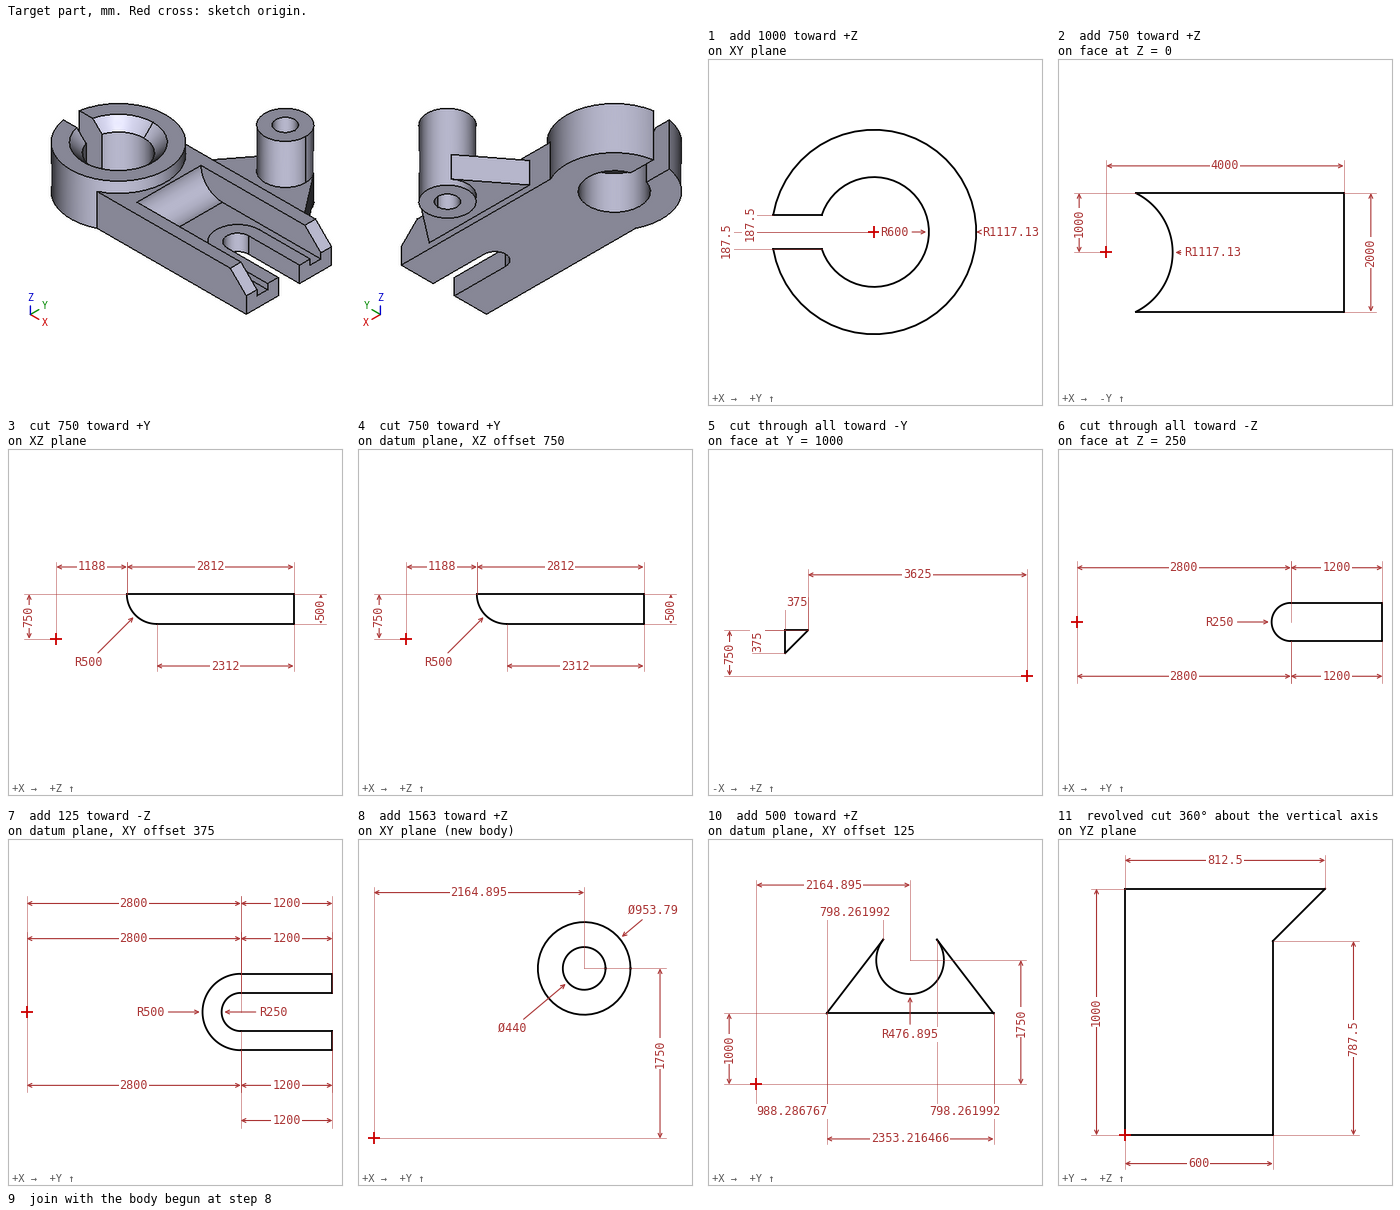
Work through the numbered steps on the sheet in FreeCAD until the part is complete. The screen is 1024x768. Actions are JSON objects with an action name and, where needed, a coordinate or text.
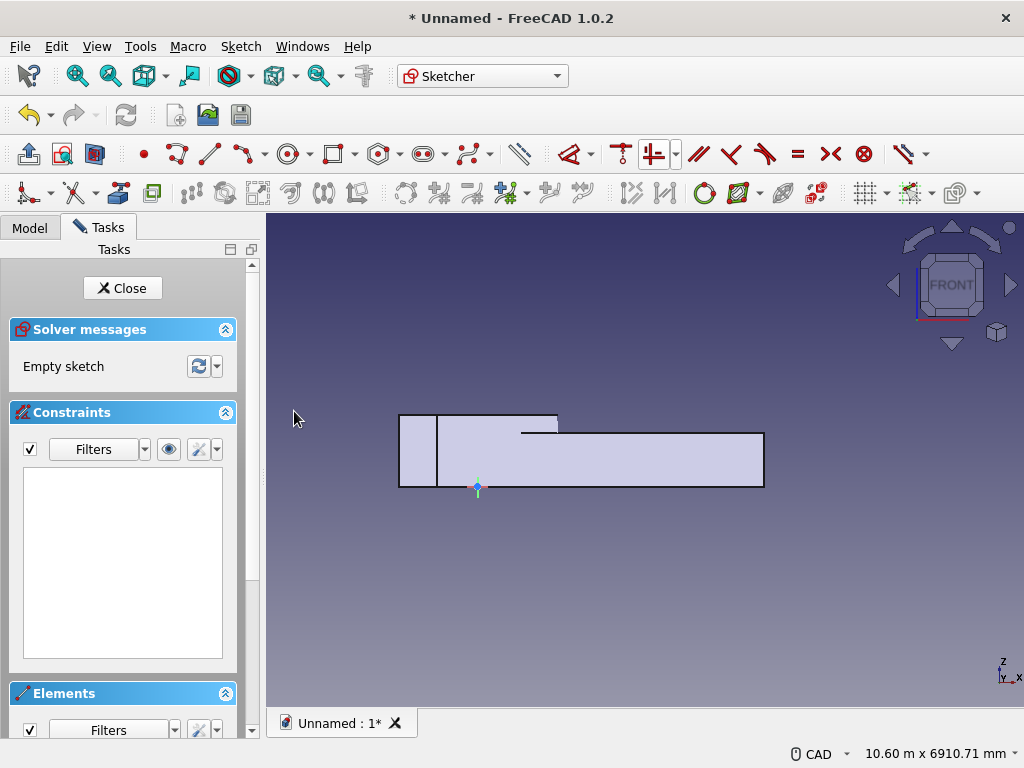
{"action": "scroll", "coordinate": [711, 460], "scroll_direction": "up", "scroll_amount": 2}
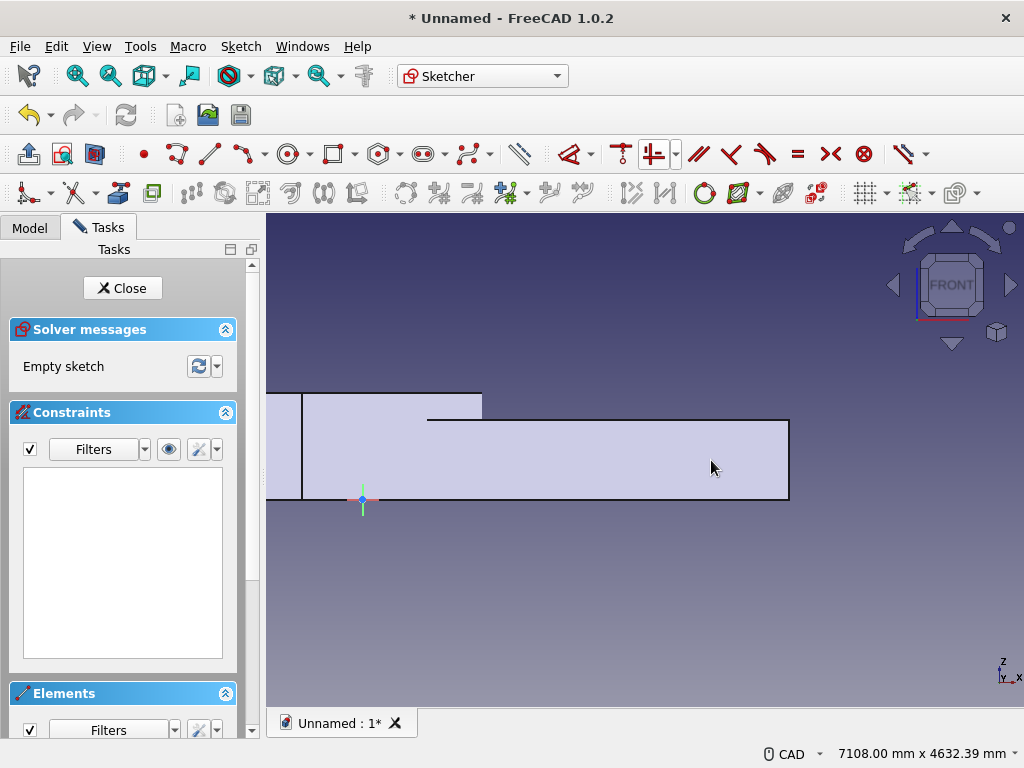
{"action": "key", "text": "g m"}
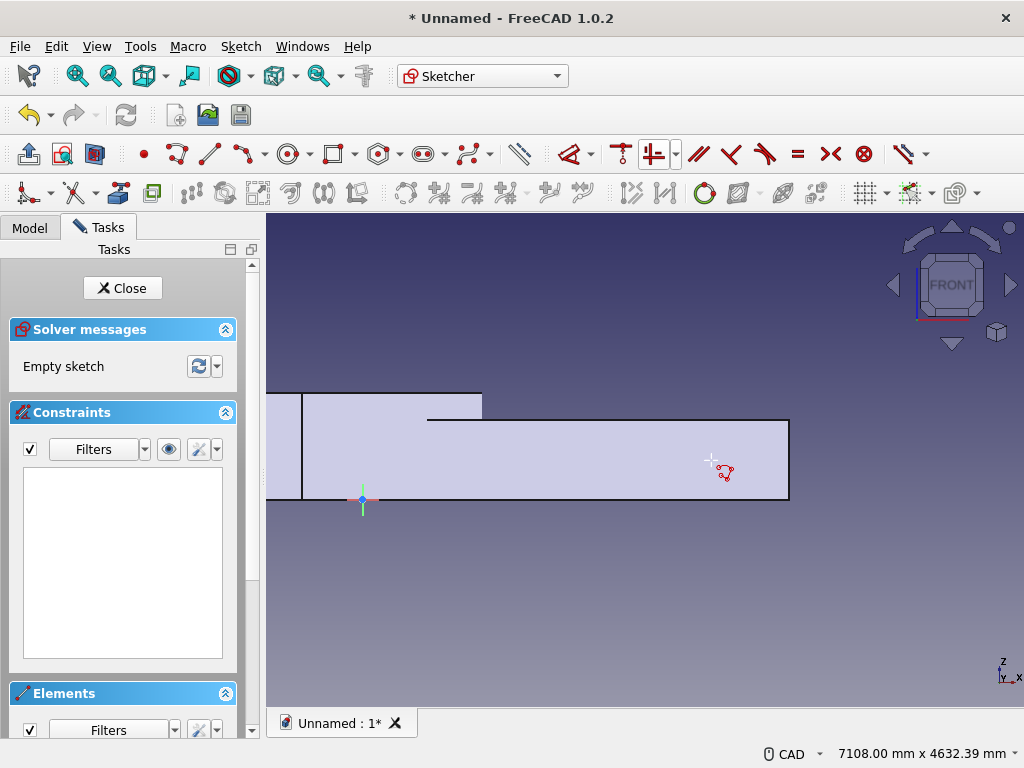
{"action": "left_click", "coordinate": [489, 420]}
{"action": "left_click", "coordinate": [789, 420]}
{"action": "left_click", "coordinate": [789, 473]}
{"action": "left_click", "coordinate": [543, 473]}
{"action": "right_click", "coordinate": [543, 473]}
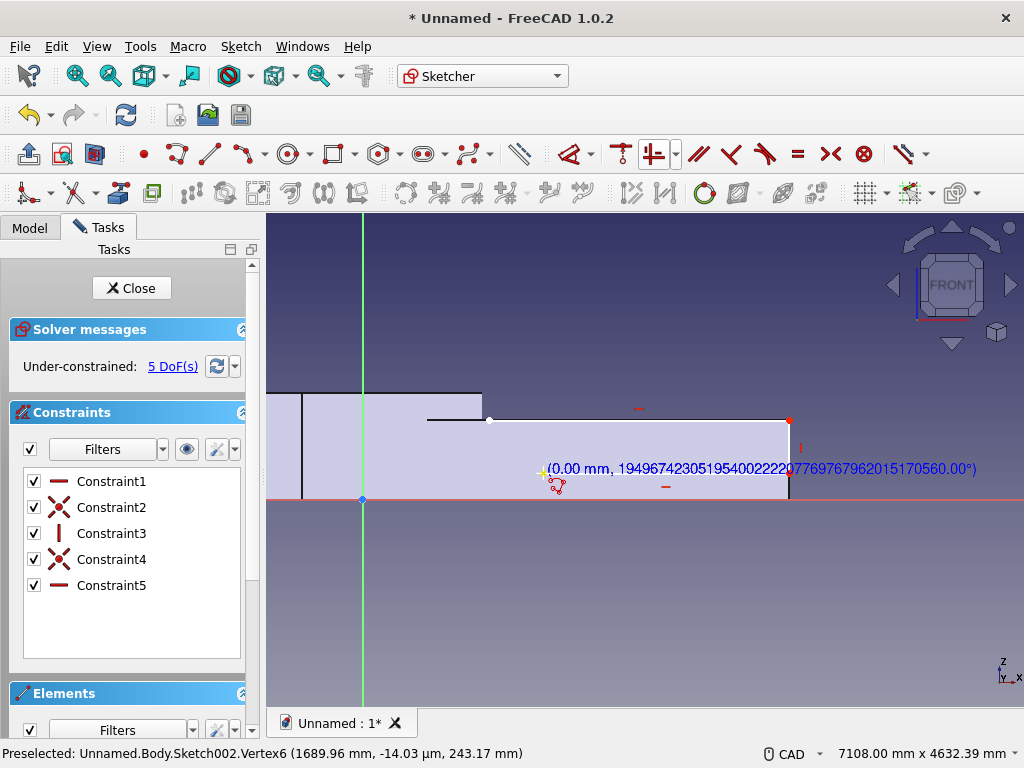
{"action": "key", "text": "g 3 a"}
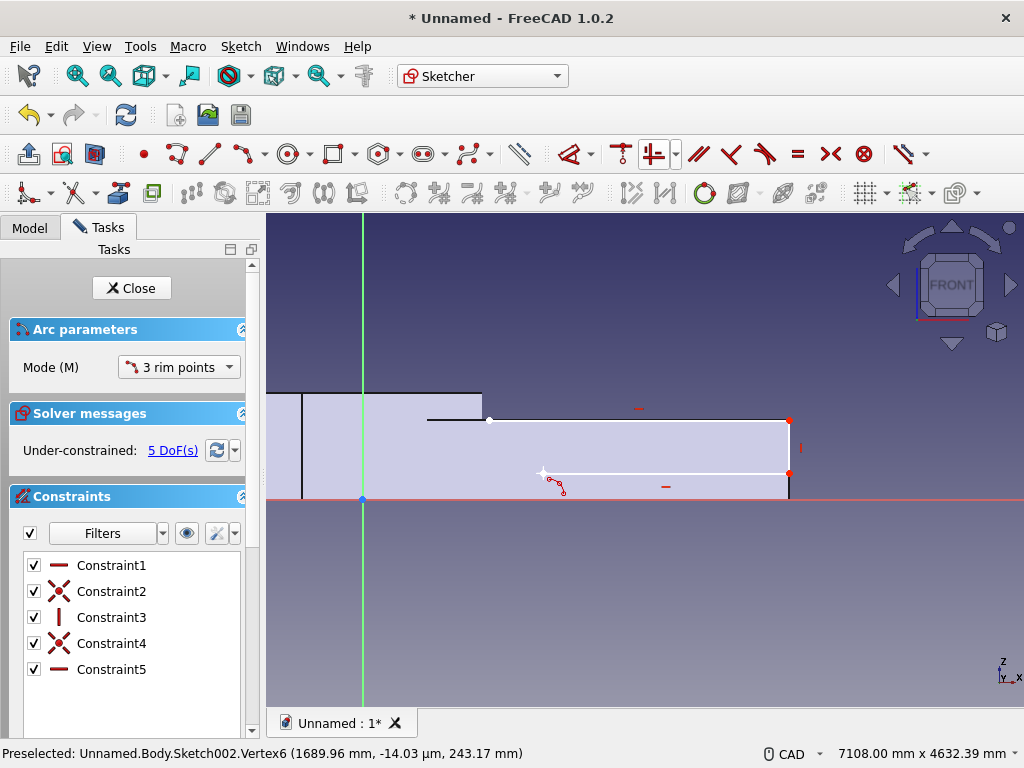
{"action": "left_click", "coordinate": [543, 474]}
{"action": "left_click", "coordinate": [489, 421]}
{"action": "left_click", "coordinate": [505, 458]}
{"action": "key", "text": "Escape"}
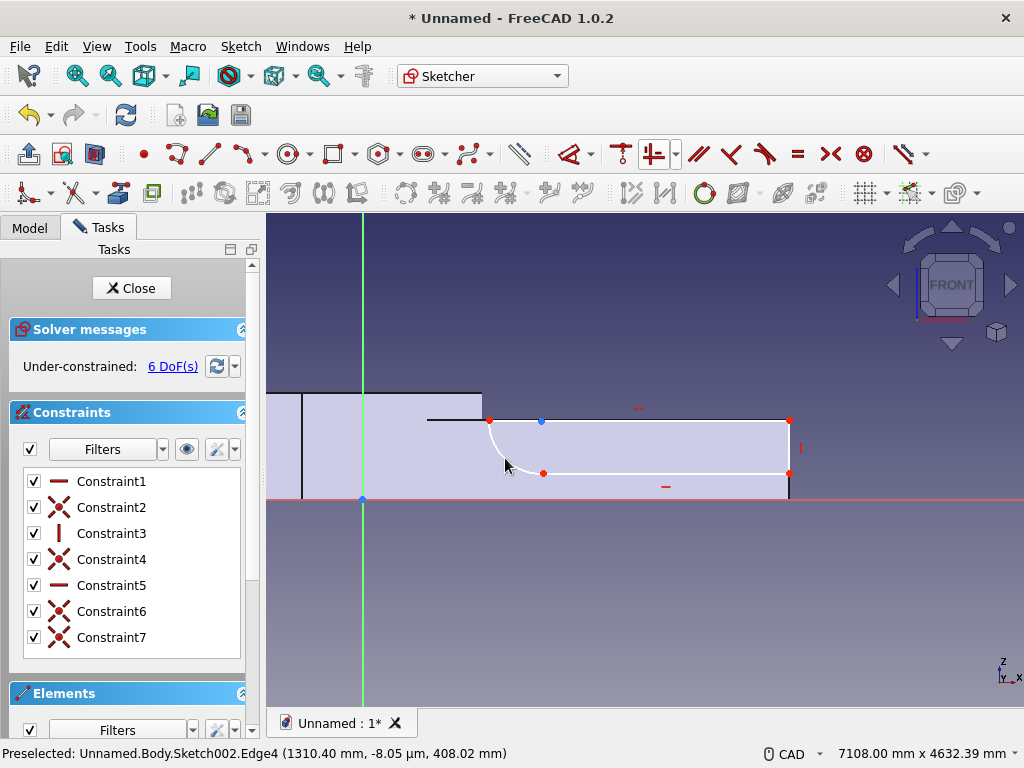
{"action": "left_click", "coordinate": [568, 154]}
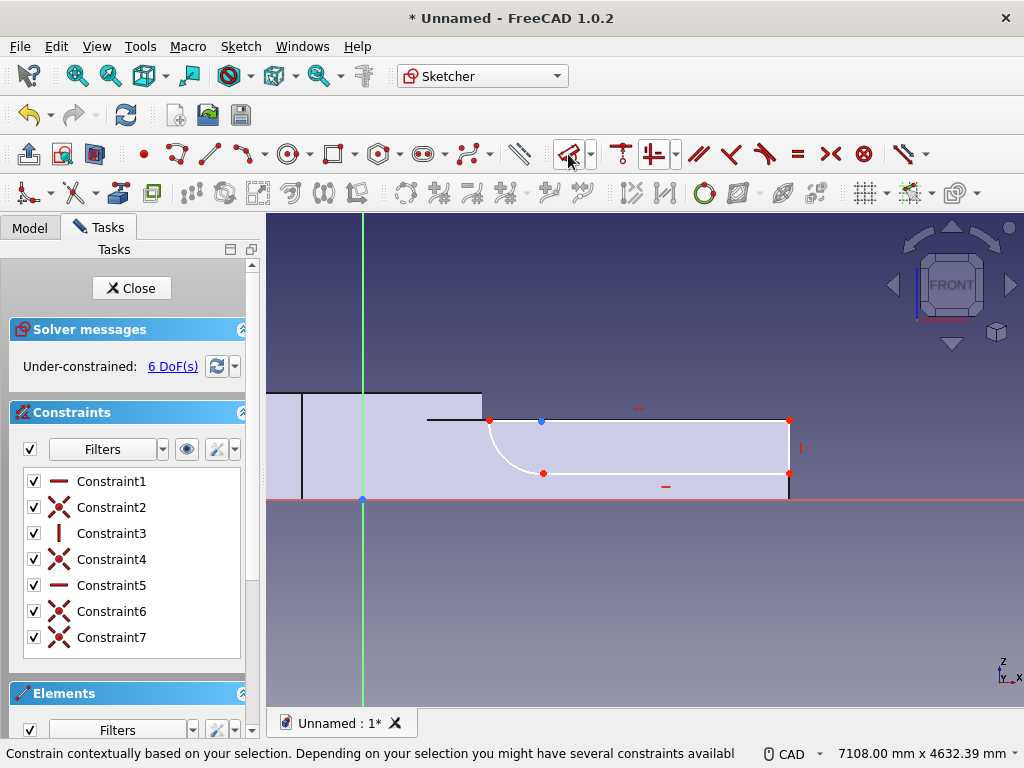
{"action": "left_click", "coordinate": [495, 445]}
{"action": "left_click", "coordinate": [466, 460]}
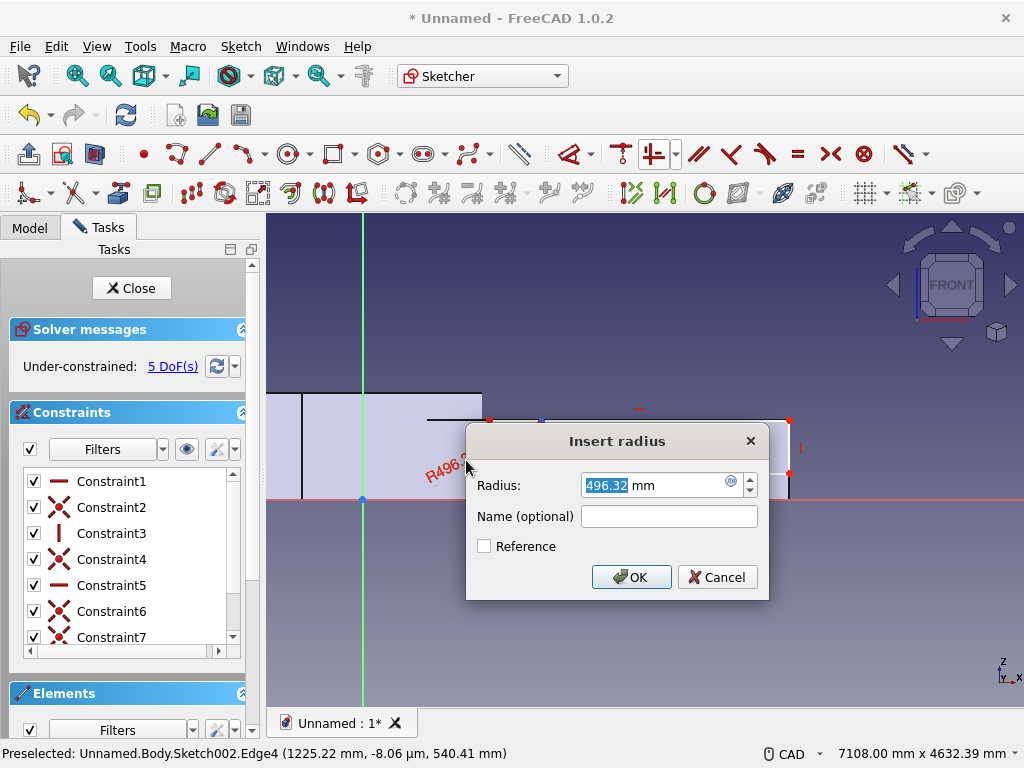
{"action": "type", "text": "500"}
{"action": "key", "text": "Return"}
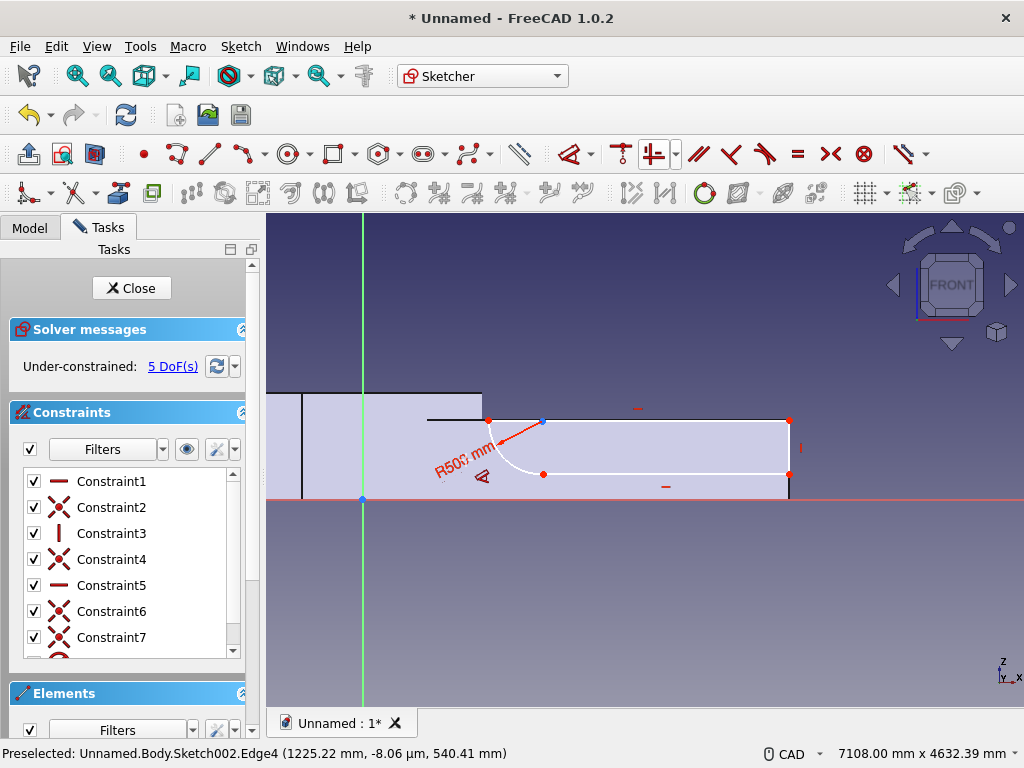
{"action": "left_click", "coordinate": [789, 437]}
{"action": "left_click", "coordinate": [823, 448]}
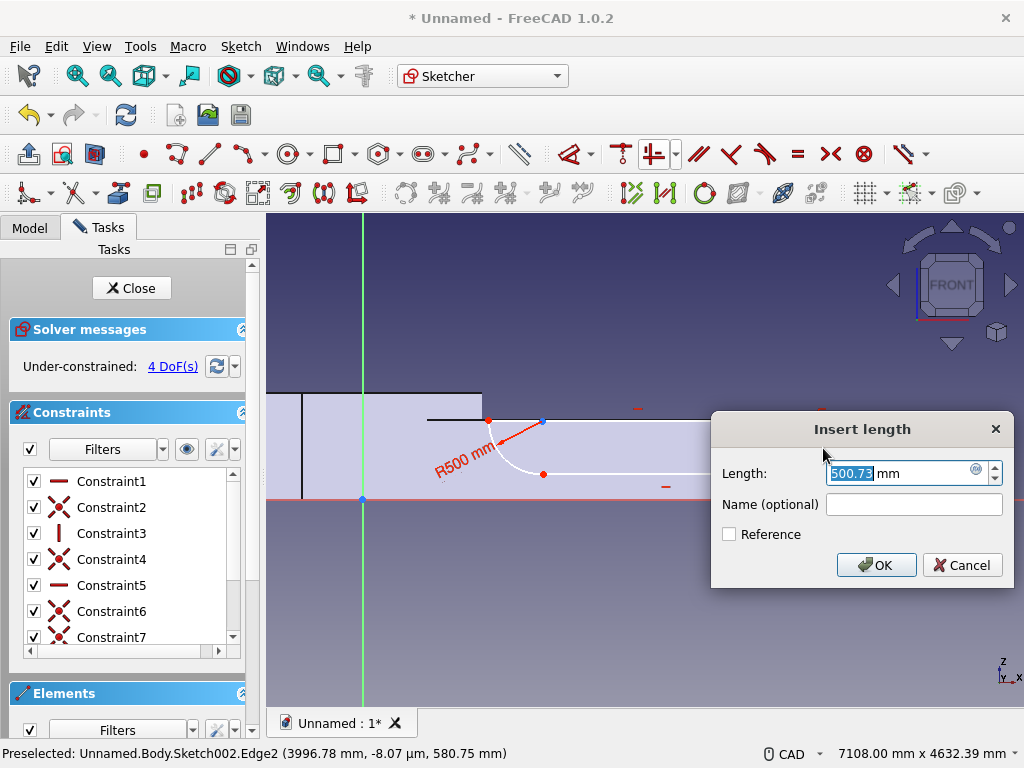
{"action": "type", "text": "500"}
{"action": "key", "text": "Return"}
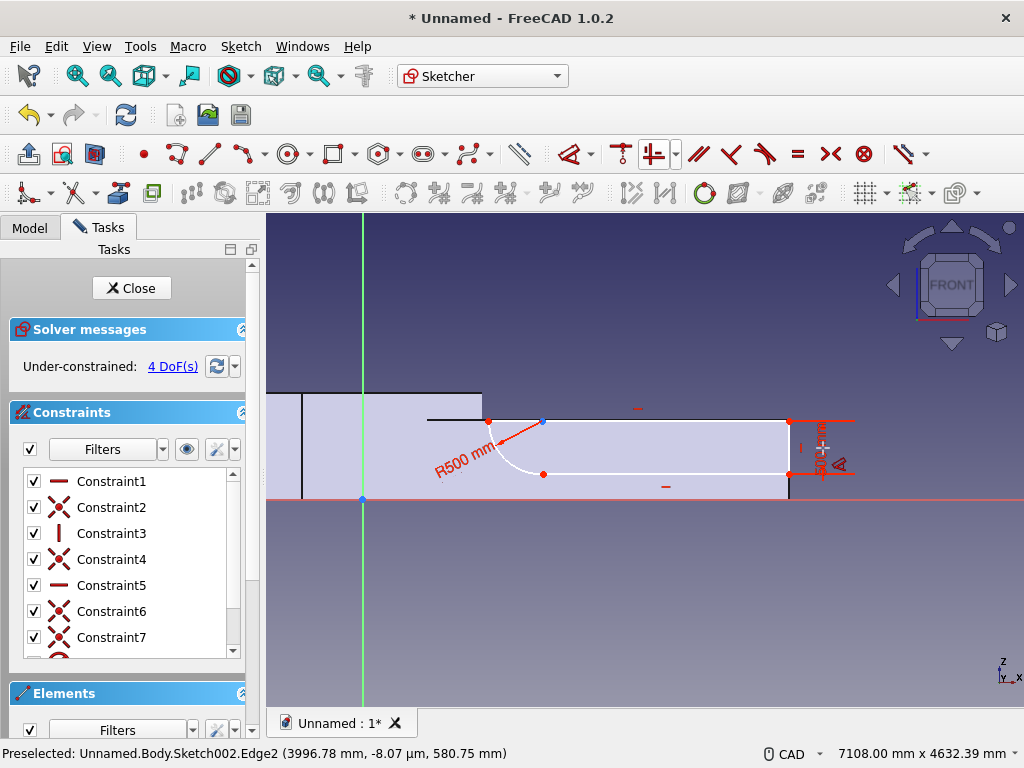
{"action": "left_click", "coordinate": [579, 421]}
{"action": "left_click", "coordinate": [639, 387]}